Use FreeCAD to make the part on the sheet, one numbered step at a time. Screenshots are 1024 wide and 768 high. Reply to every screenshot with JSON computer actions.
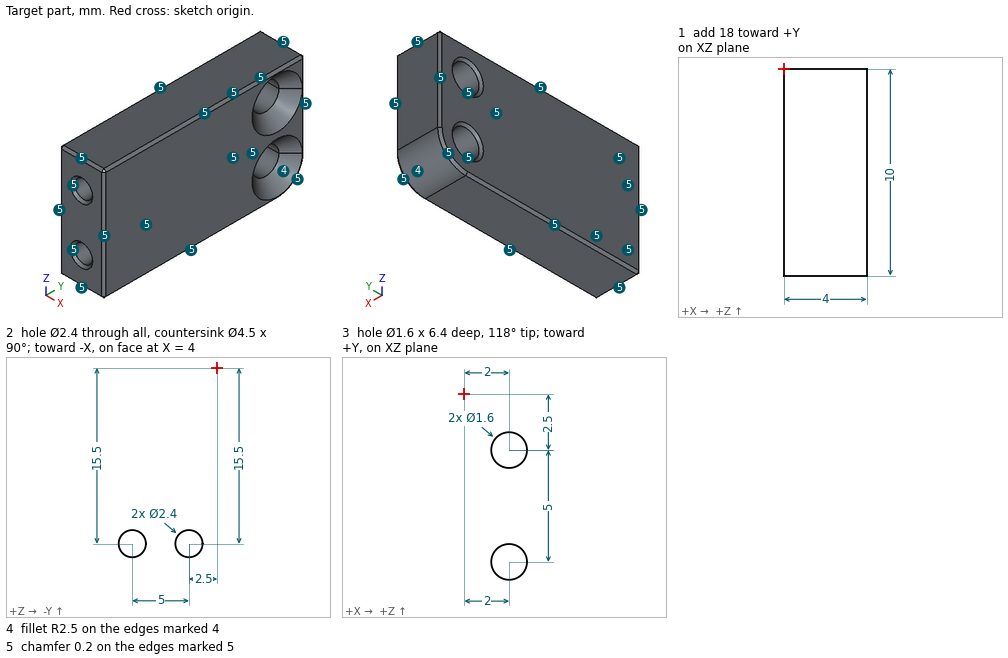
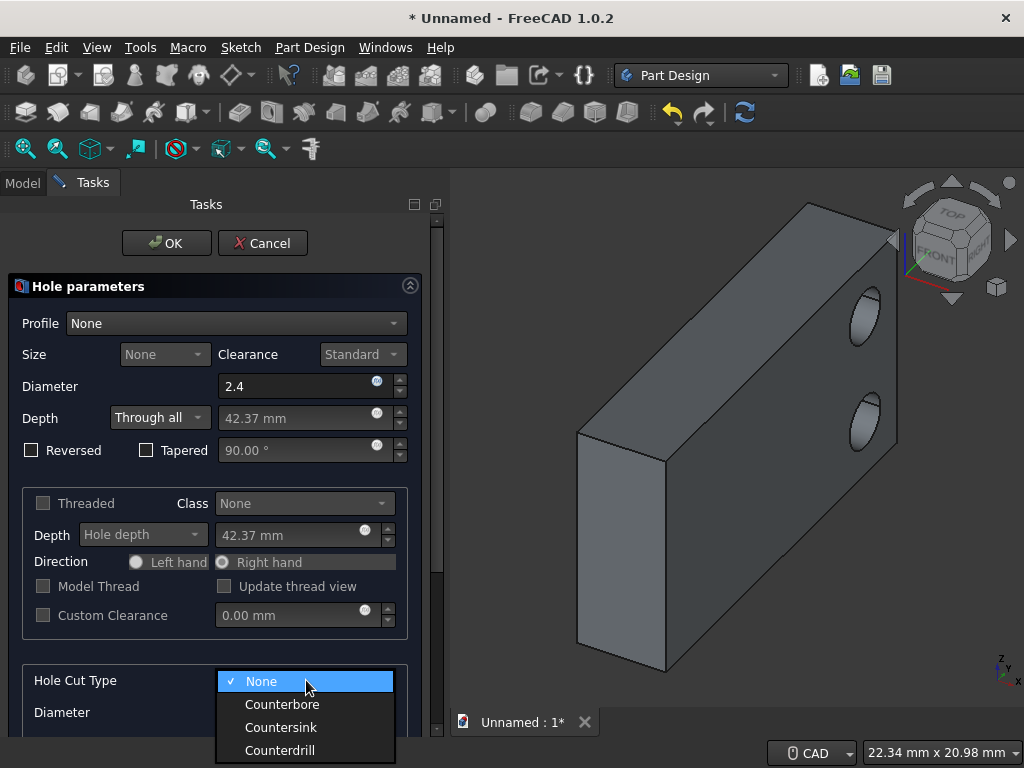
{"action": "left_click", "coordinate": [304, 728]}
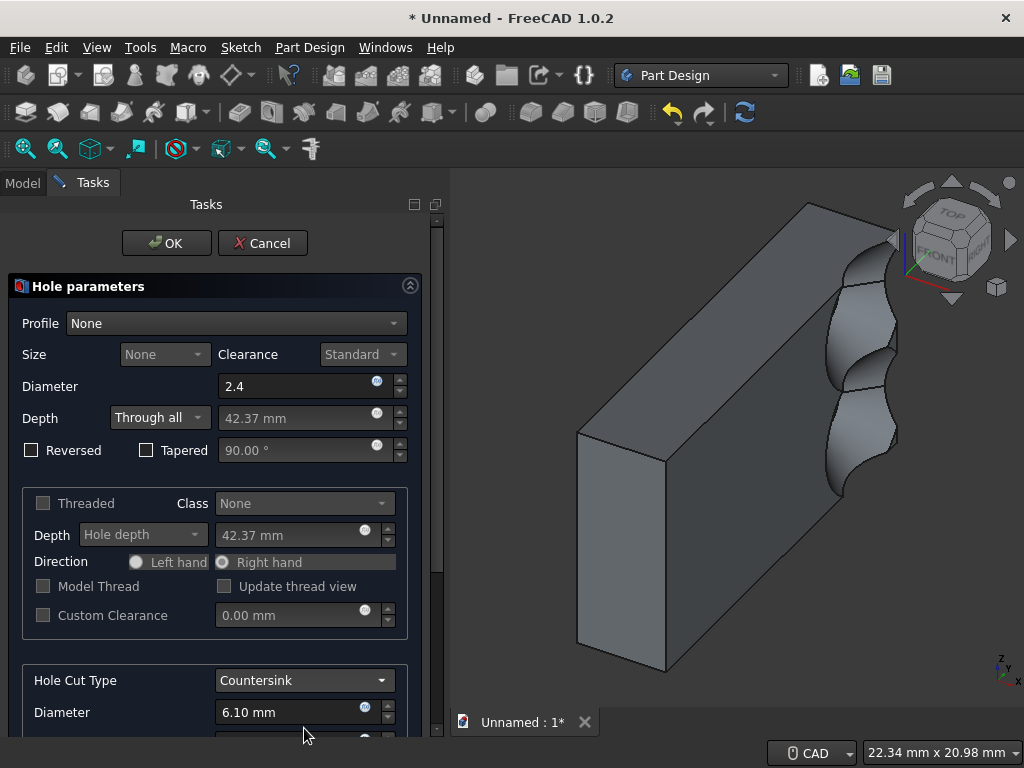
{"action": "triple_click", "coordinate": [298, 712]}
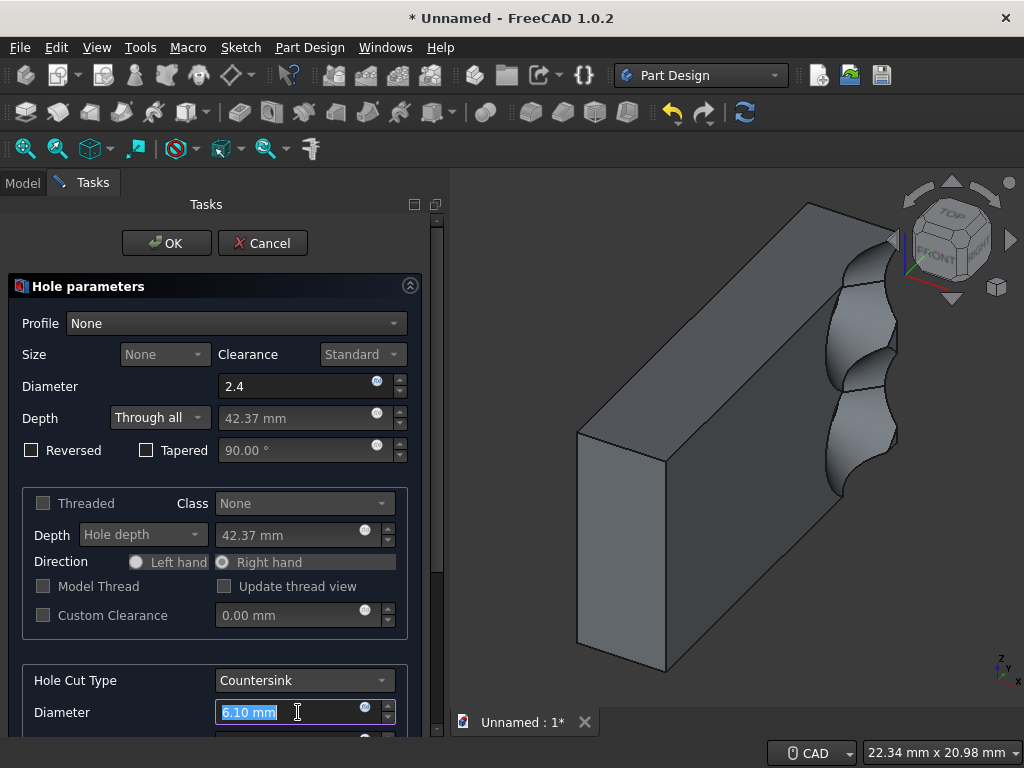
{"action": "type", "text": "4.5"}
{"action": "key", "text": "Tab"}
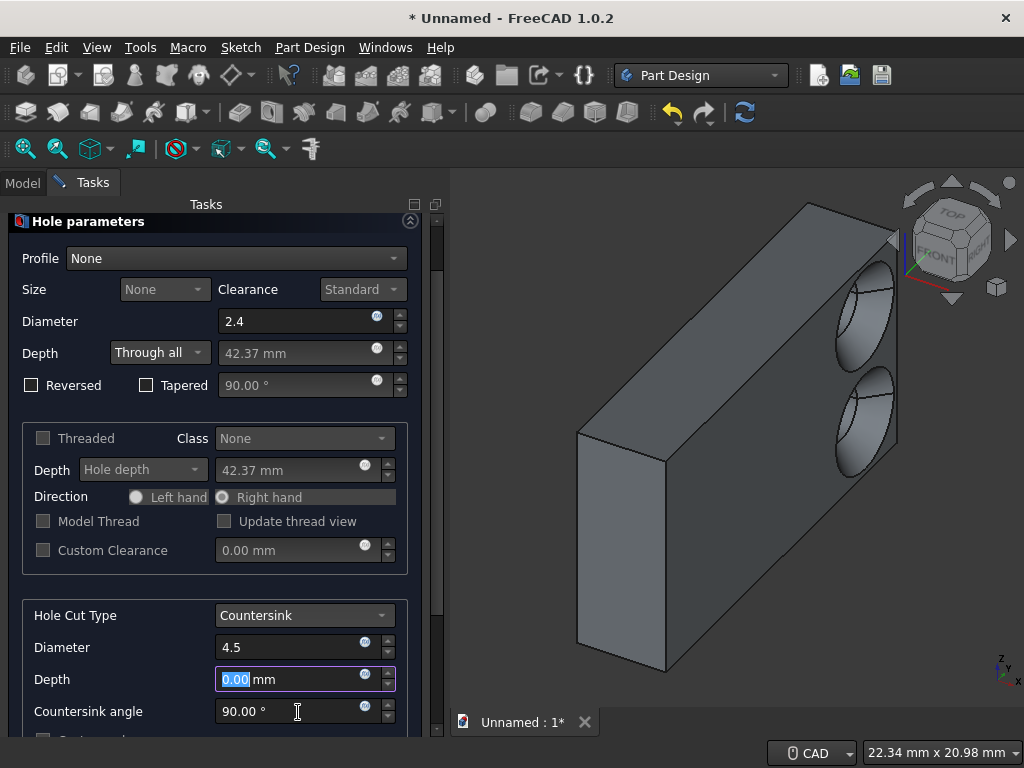
{"action": "scroll", "coordinate": [437, 475], "scroll_direction": "up", "scroll_amount": 2}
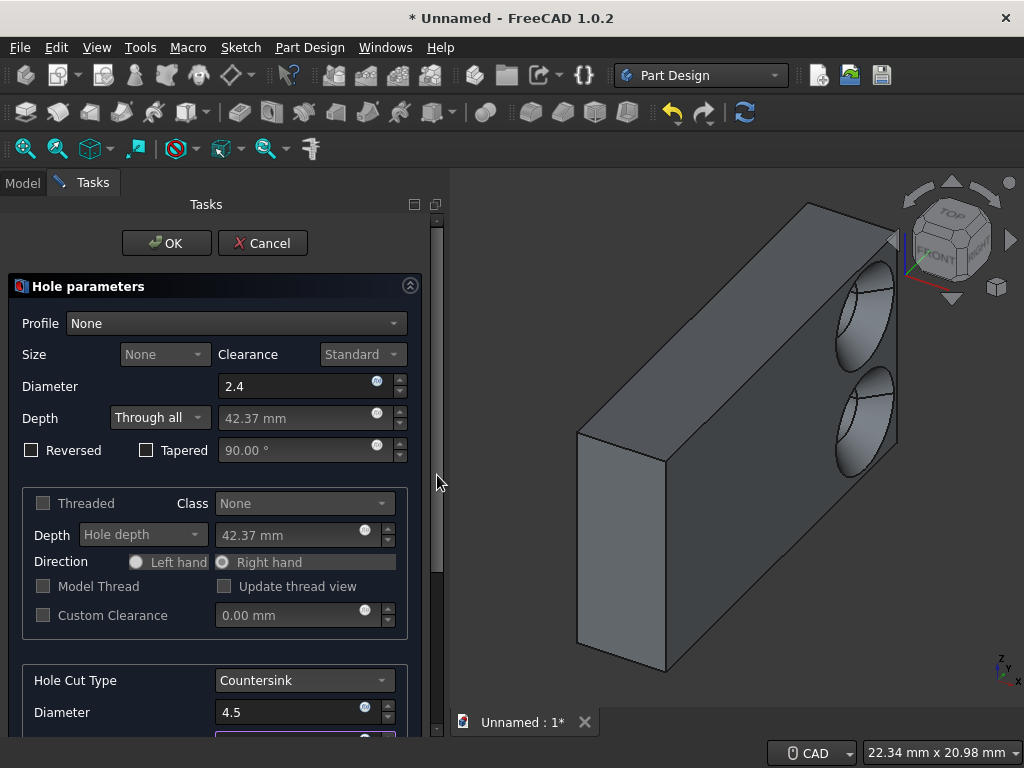
{"action": "left_click", "coordinate": [167, 243]}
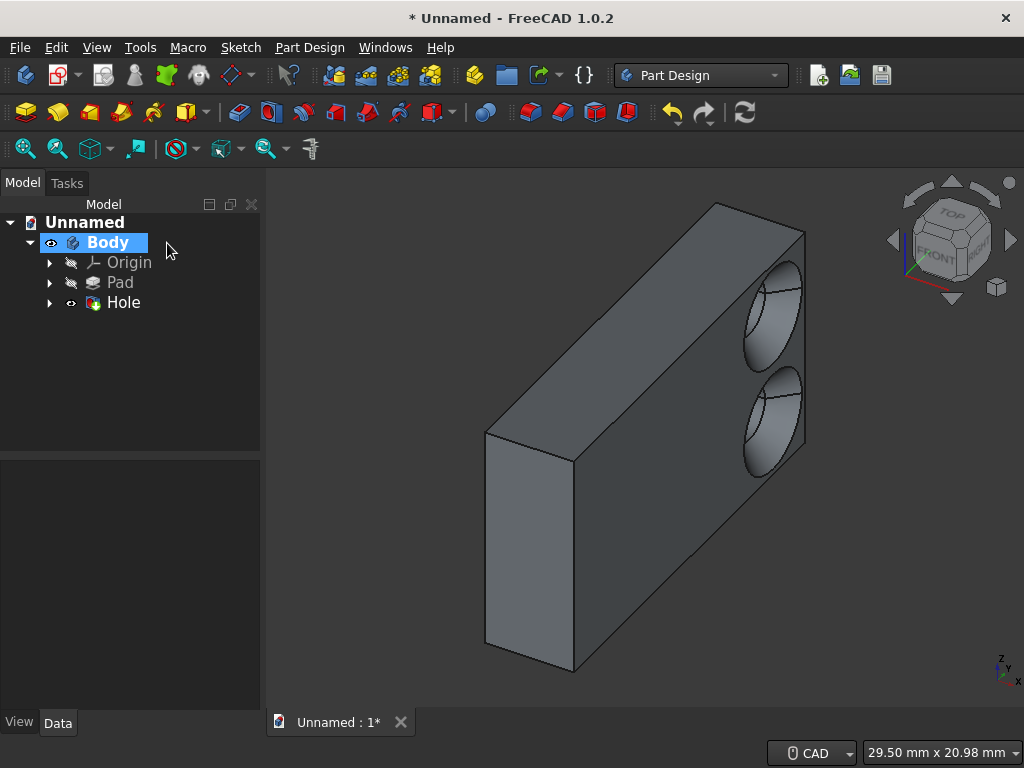
{"action": "left_click", "coordinate": [58, 76]}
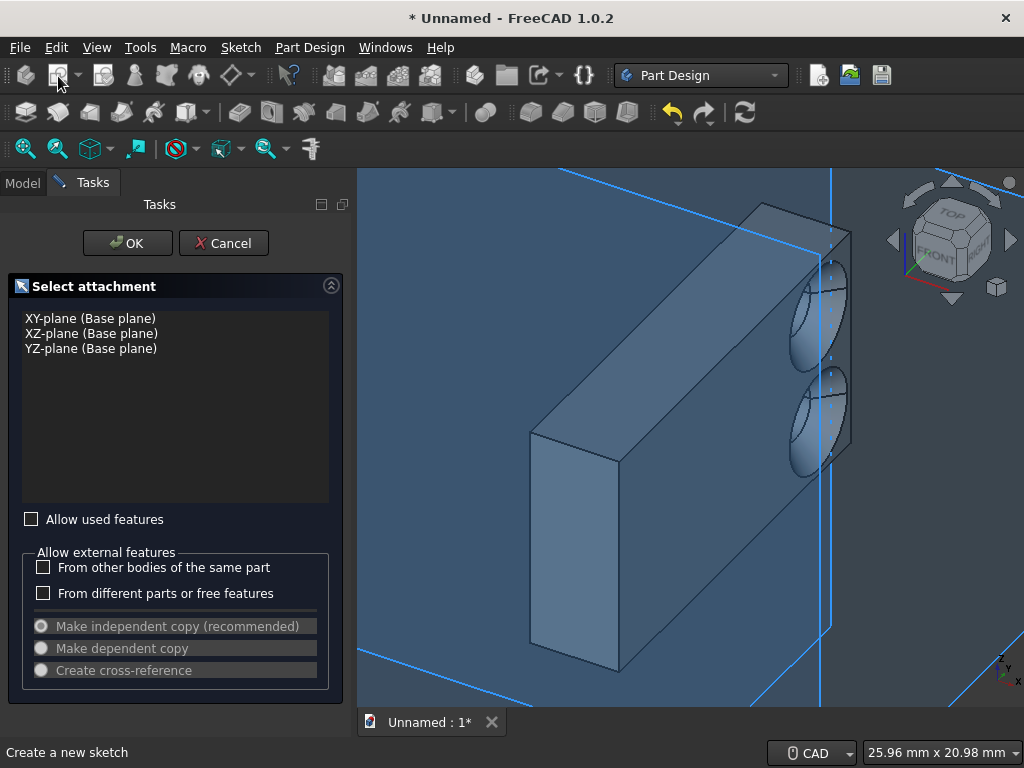
{"action": "left_click", "coordinate": [82, 334]}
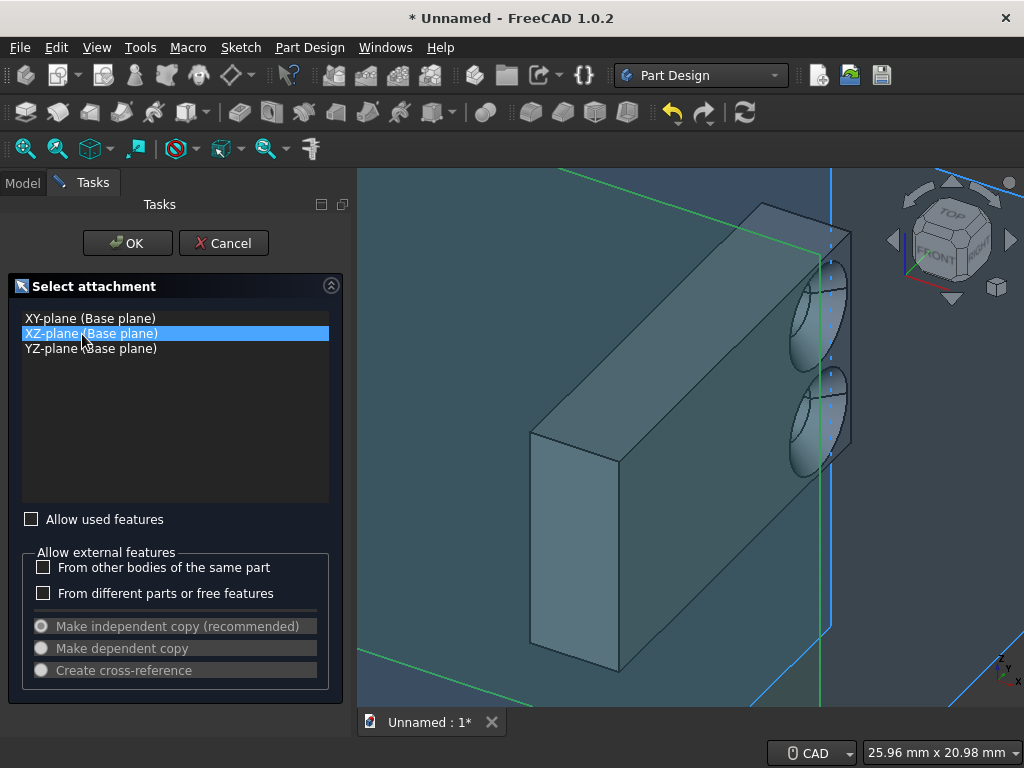
{"action": "left_click", "coordinate": [128, 243]}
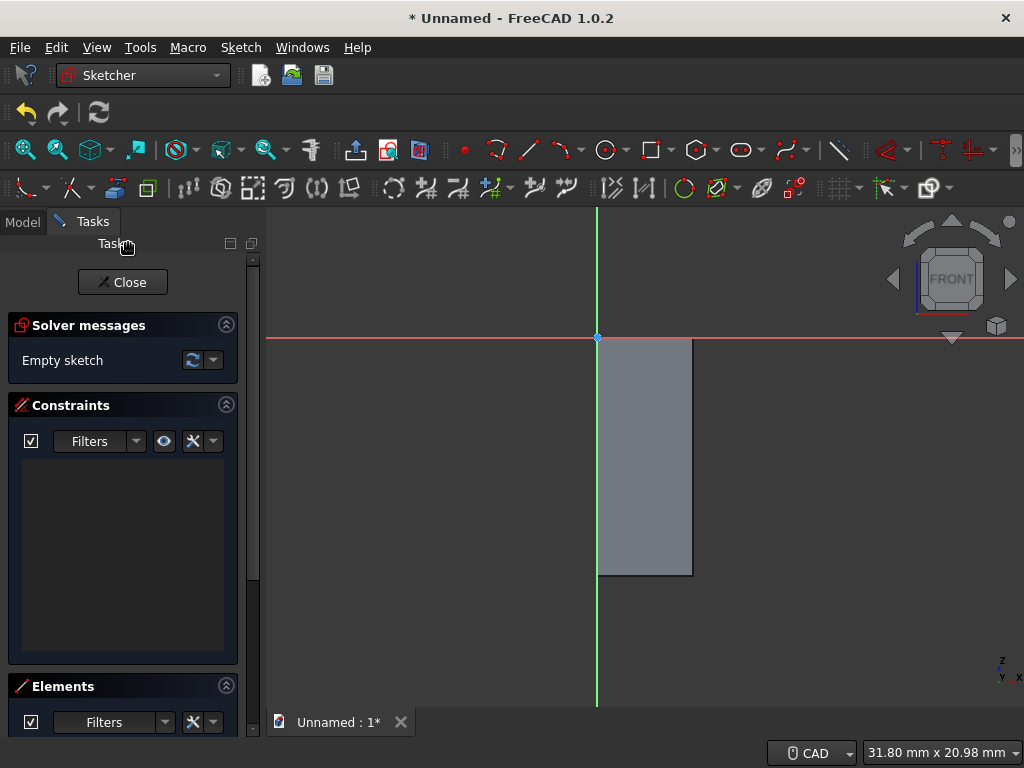
{"action": "scroll", "coordinate": [741, 396], "scroll_direction": "up", "scroll_amount": 2}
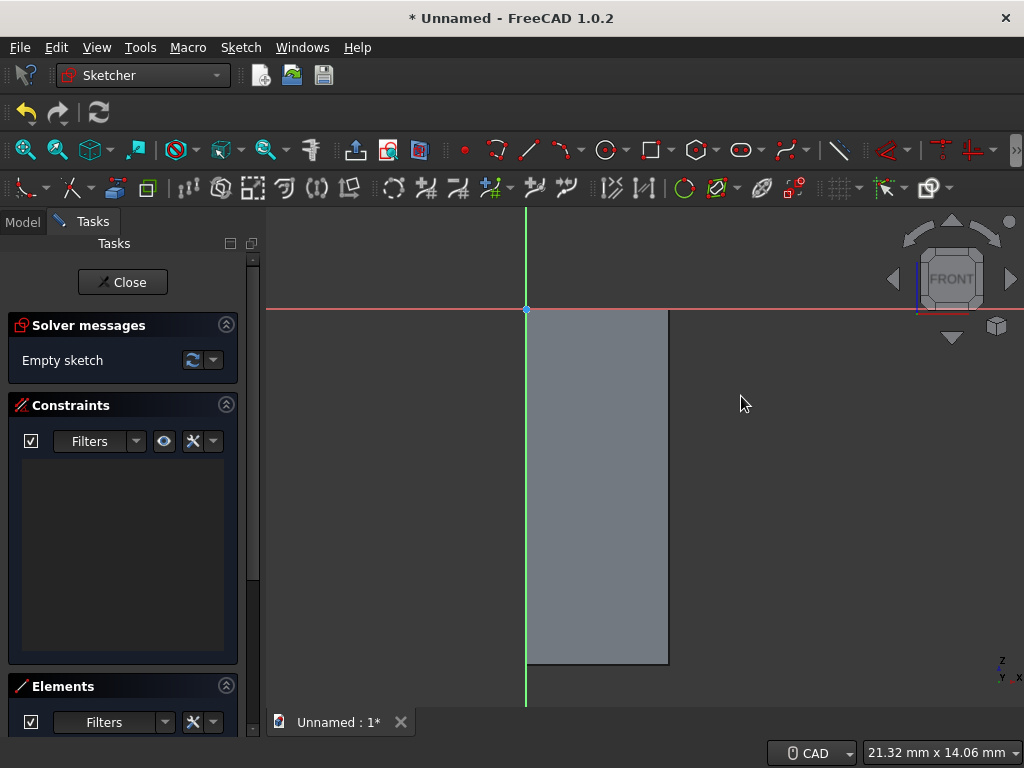
{"action": "left_click", "coordinate": [606, 150]}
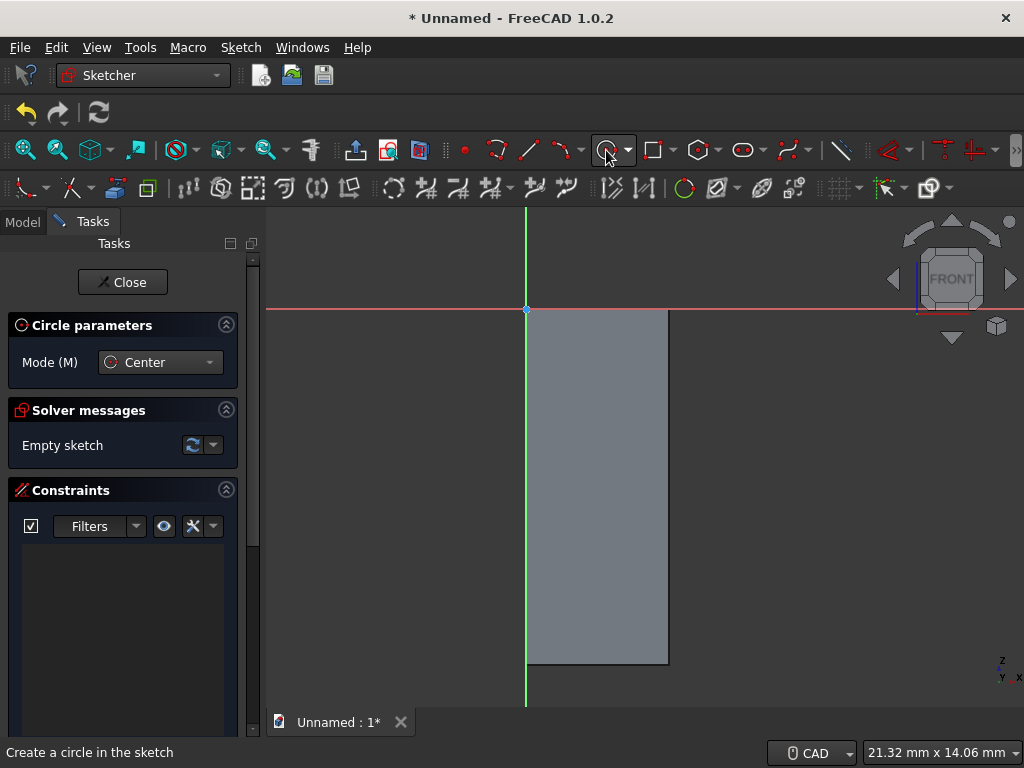
{"action": "left_click", "coordinate": [597, 398]}
{"action": "mouse_move", "coordinate": [618, 378]}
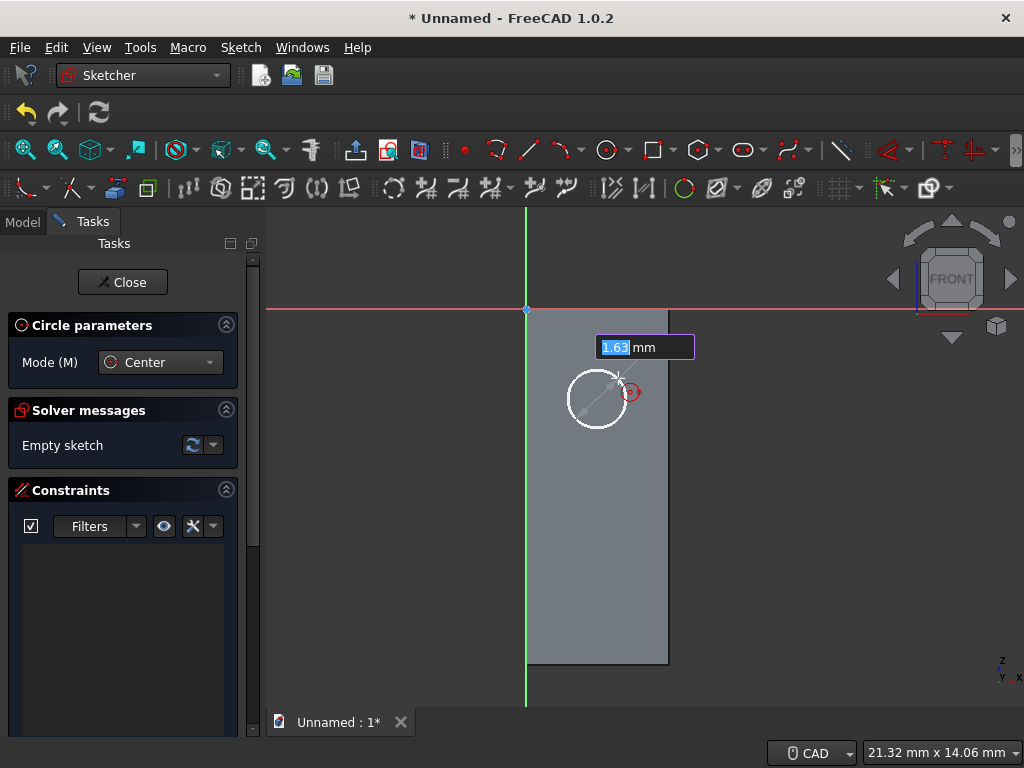
{"action": "type", "text": "1.6"}
{"action": "key", "text": "Return"}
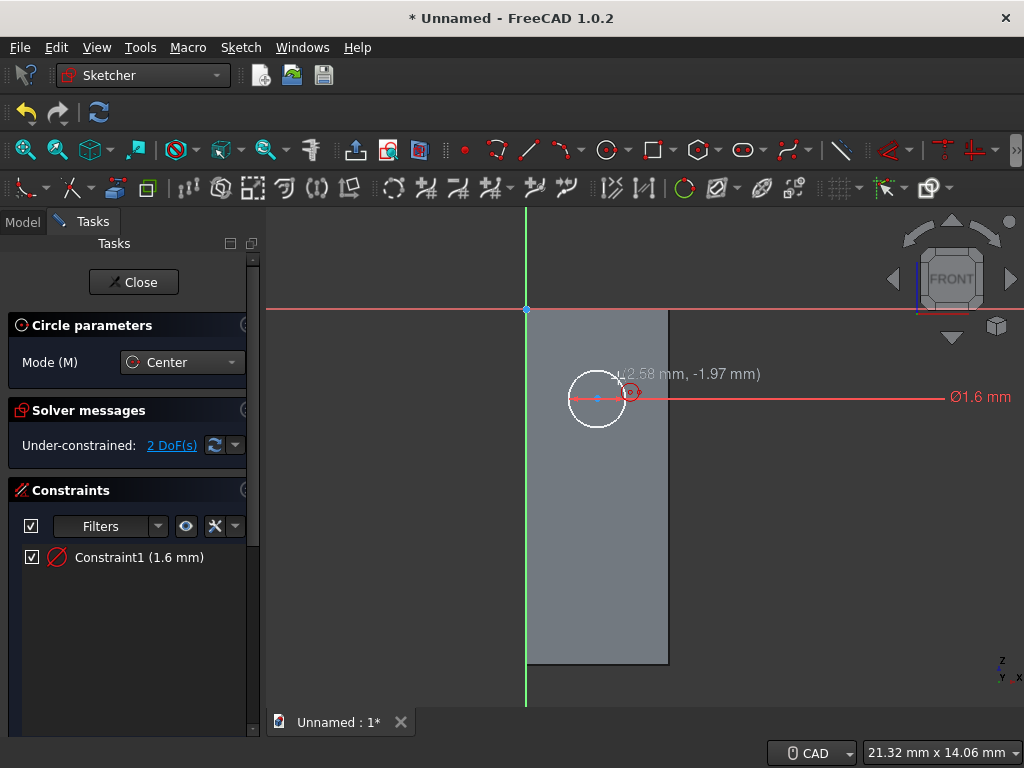
{"action": "left_click", "coordinate": [597, 576]}
{"action": "mouse_move", "coordinate": [618, 556]}